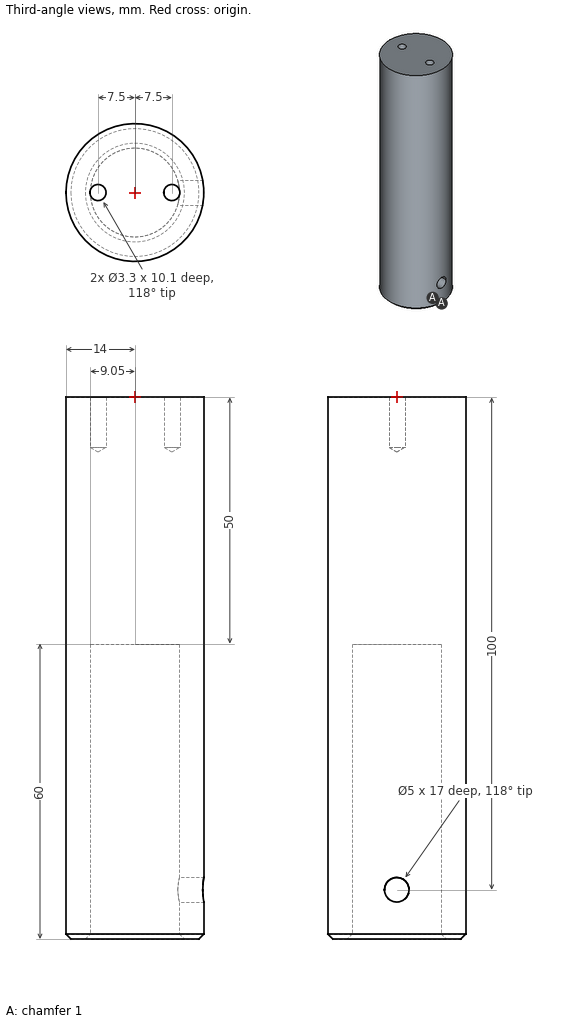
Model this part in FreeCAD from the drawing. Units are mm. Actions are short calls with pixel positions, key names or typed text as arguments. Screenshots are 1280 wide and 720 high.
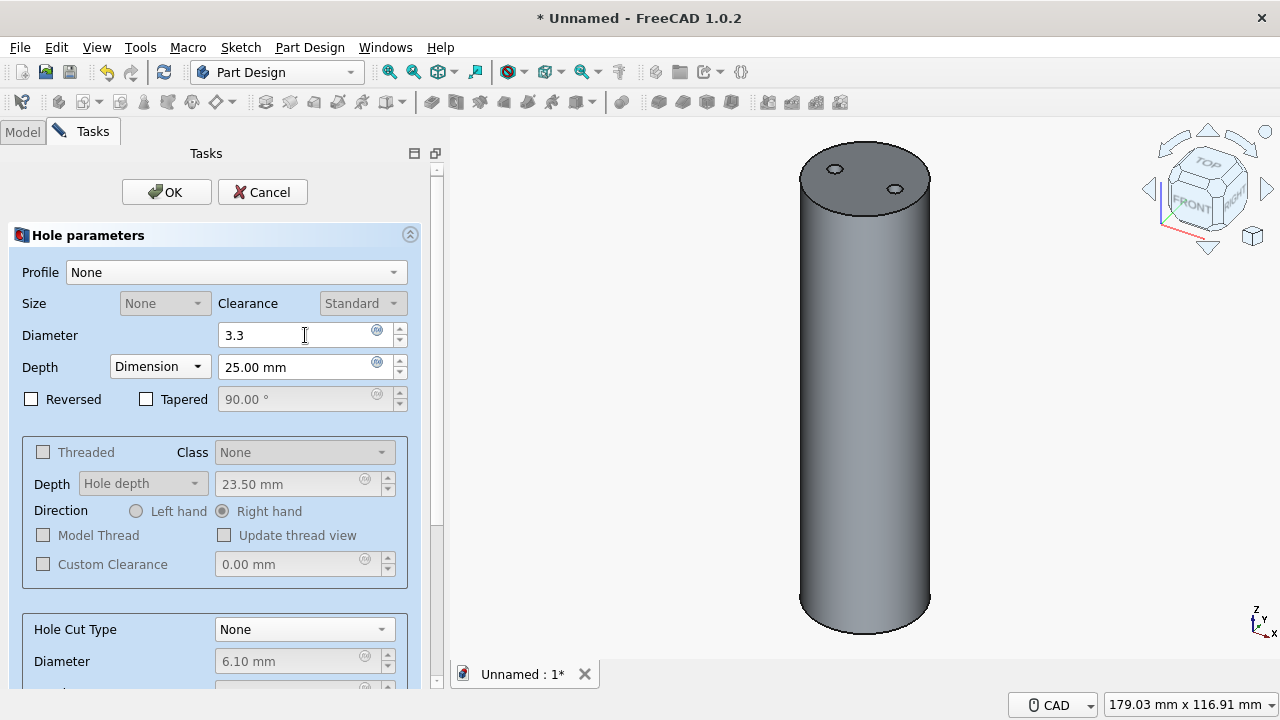
triple_click(305, 367)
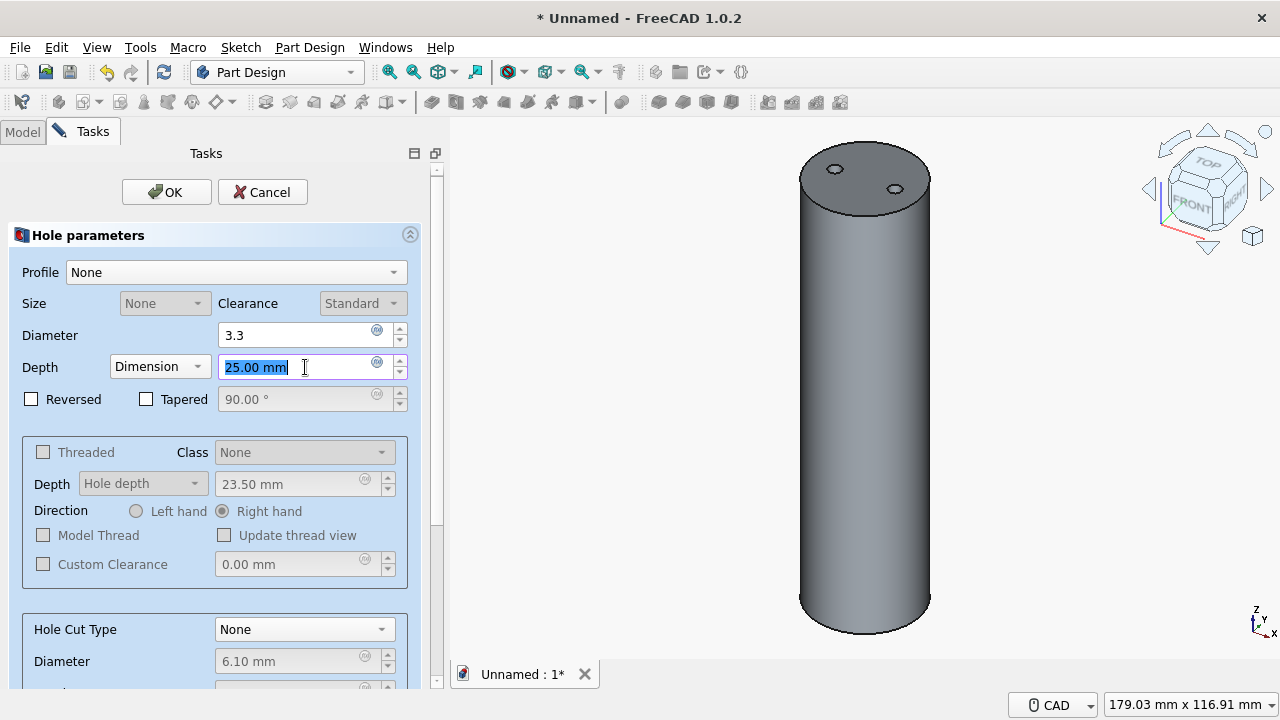
text(10.1)
key(Tab)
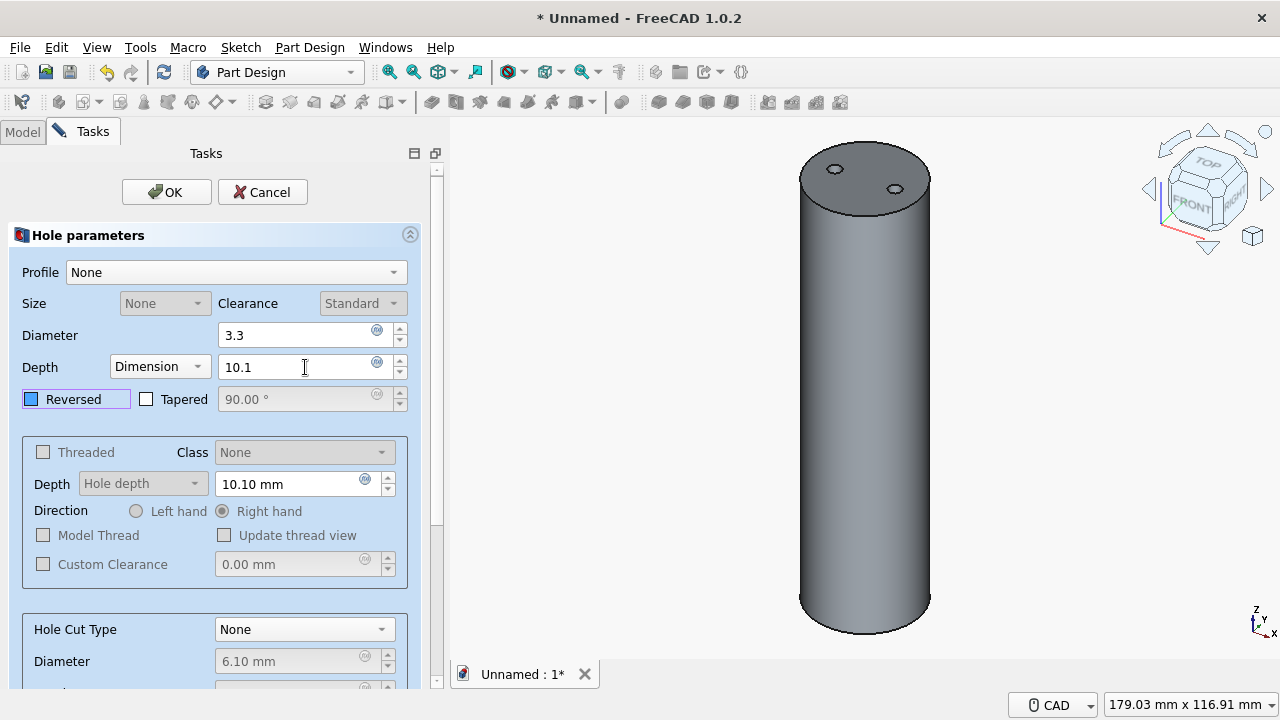
click(167, 192)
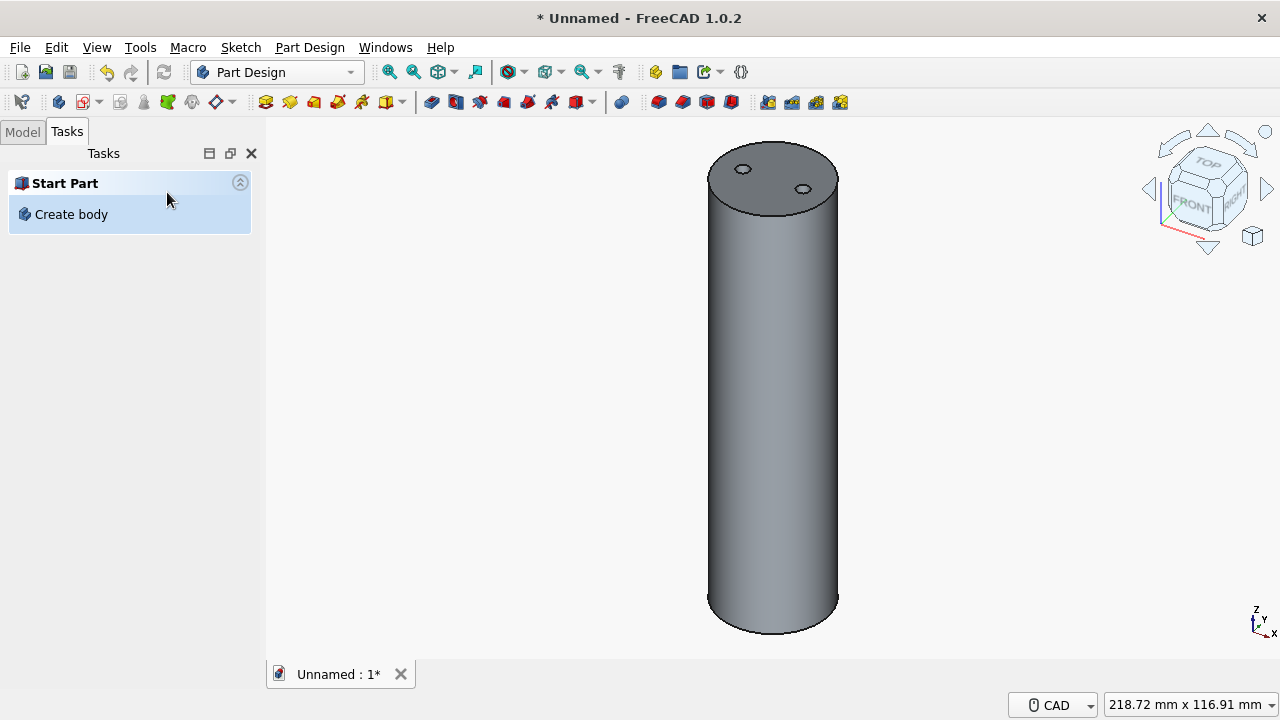
click(23, 131)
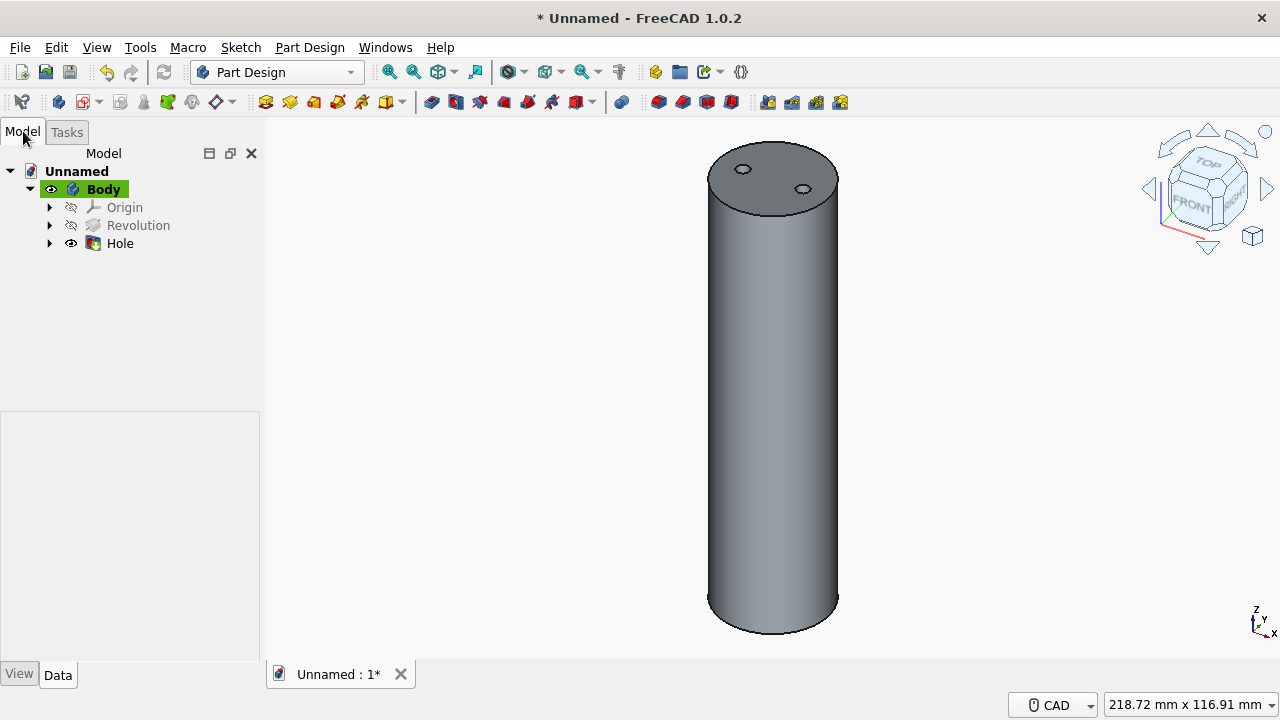
click(50, 207)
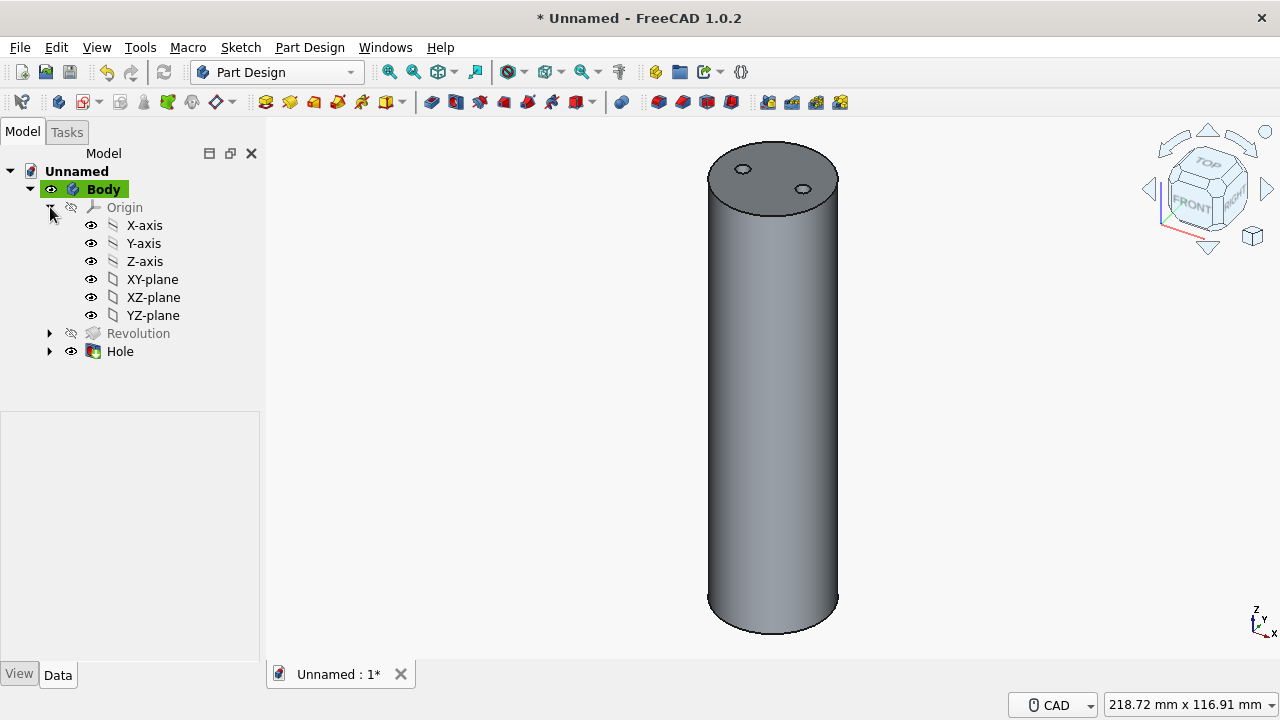
click(136, 315)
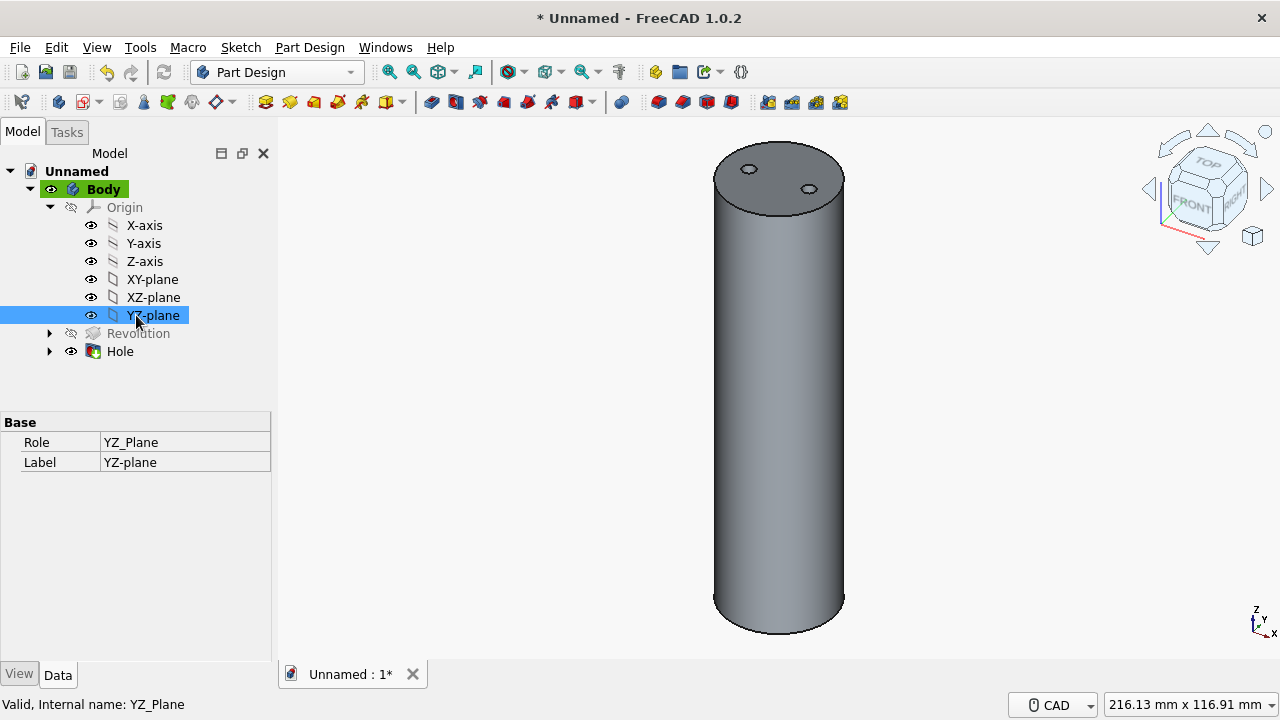
click(216, 102)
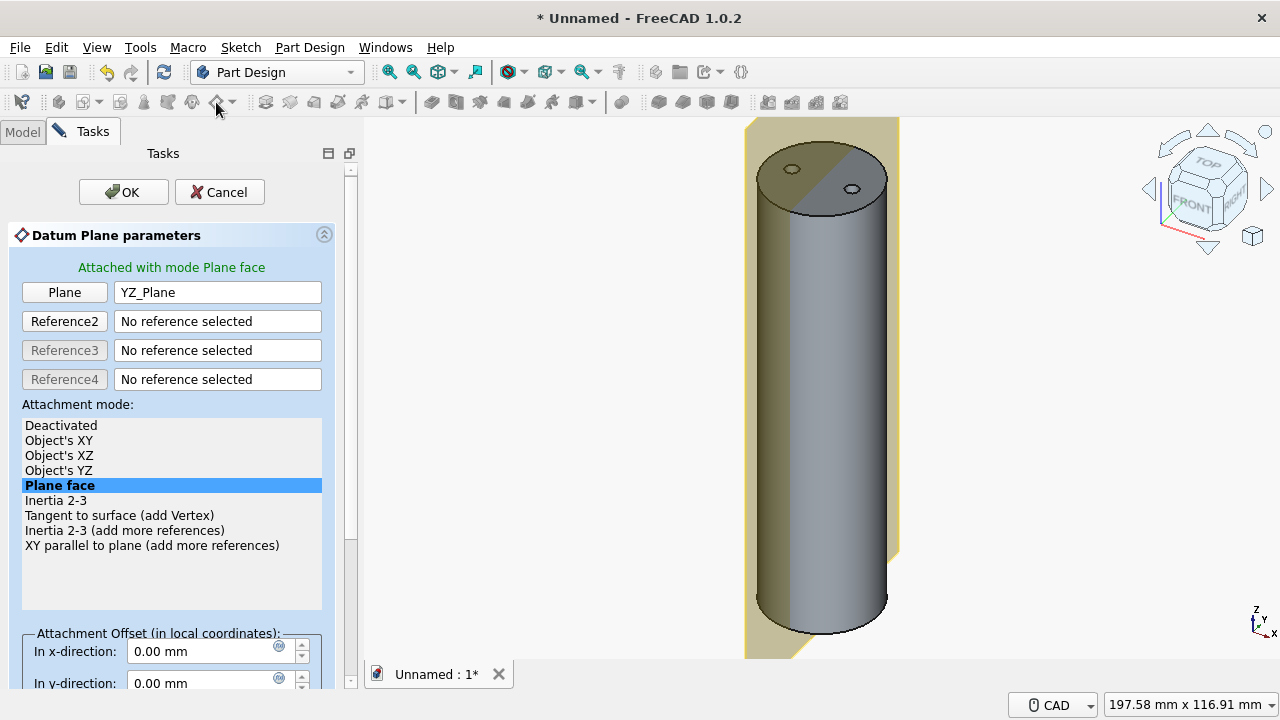
scroll(351, 426, down, 2)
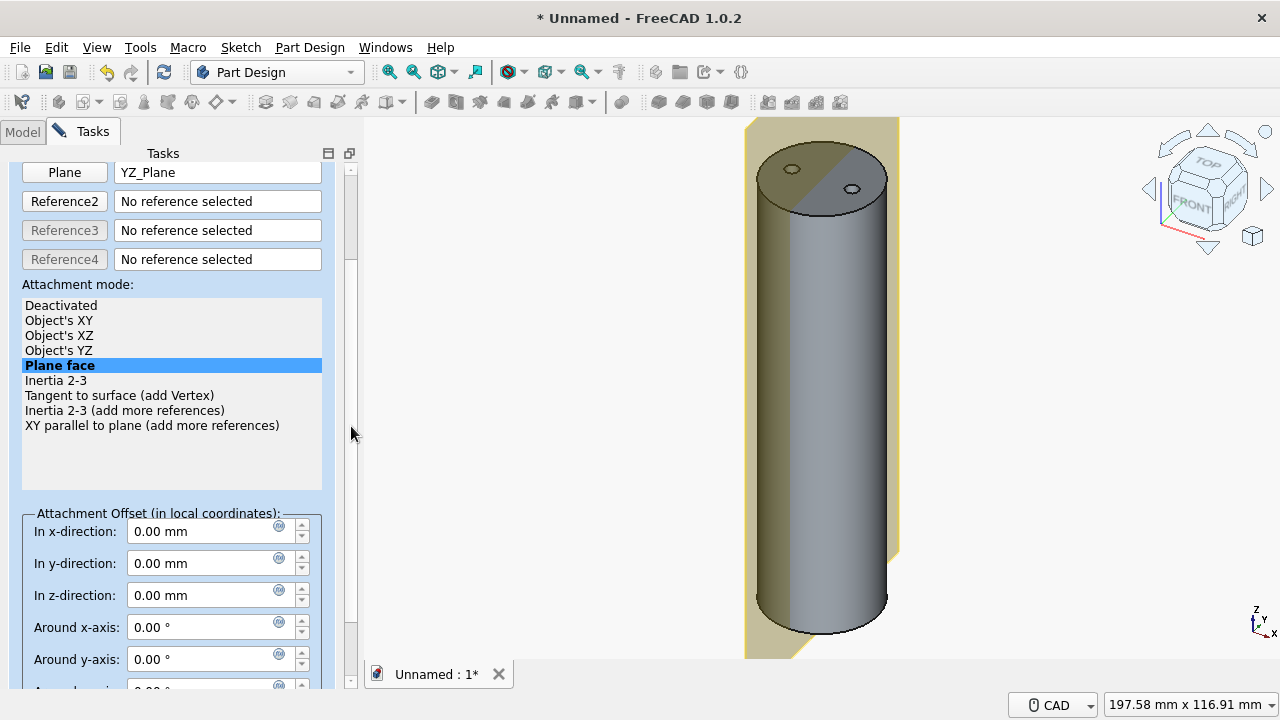
triple_click(210, 595)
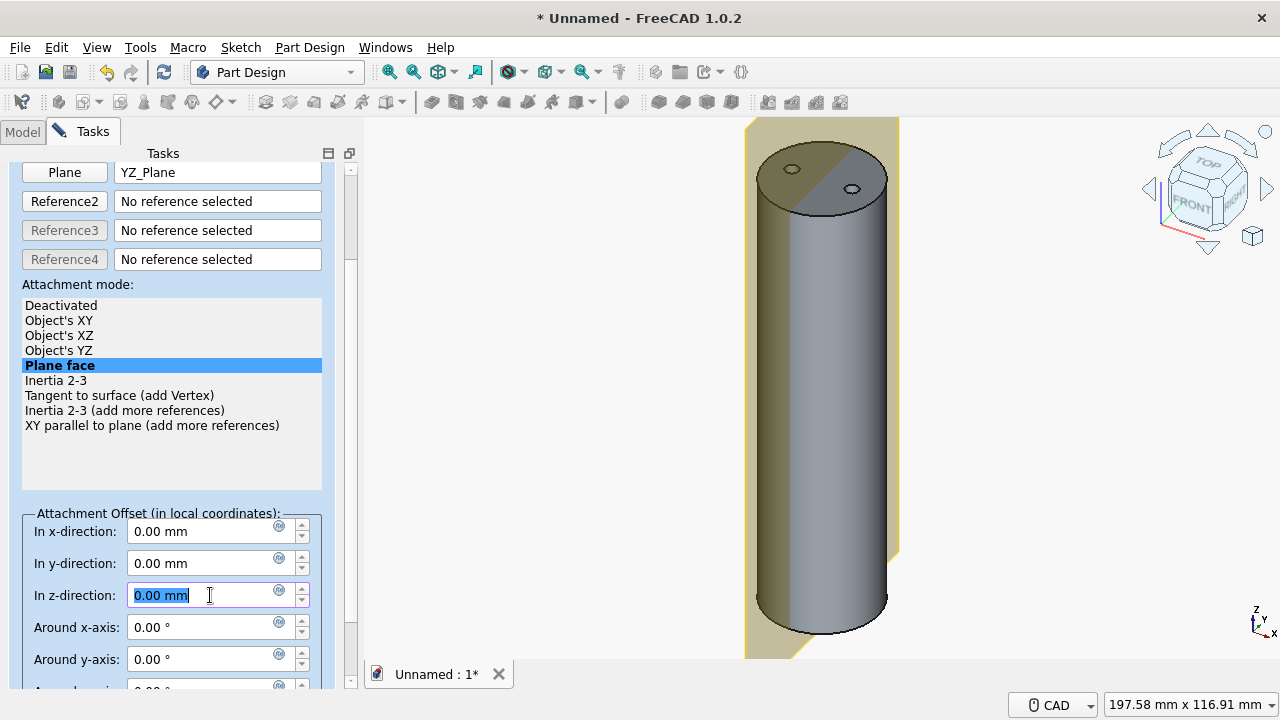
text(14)
key(Tab)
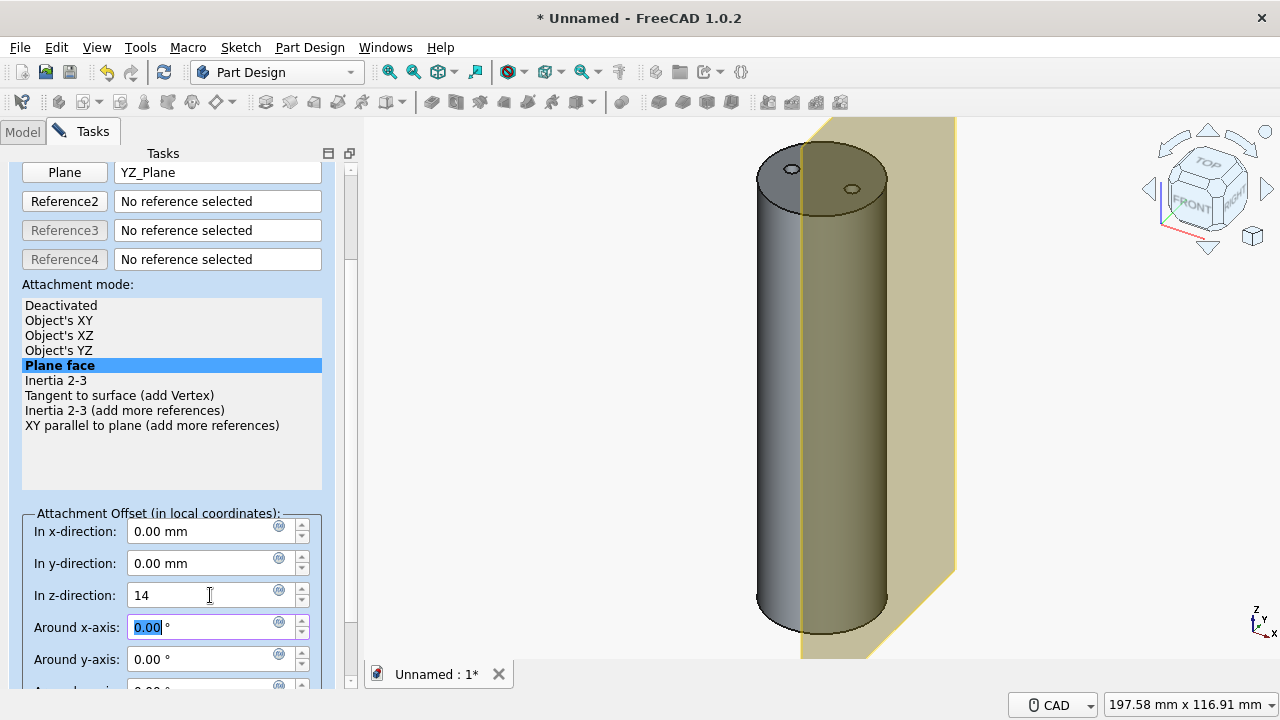
scroll(351, 426, up, 3)